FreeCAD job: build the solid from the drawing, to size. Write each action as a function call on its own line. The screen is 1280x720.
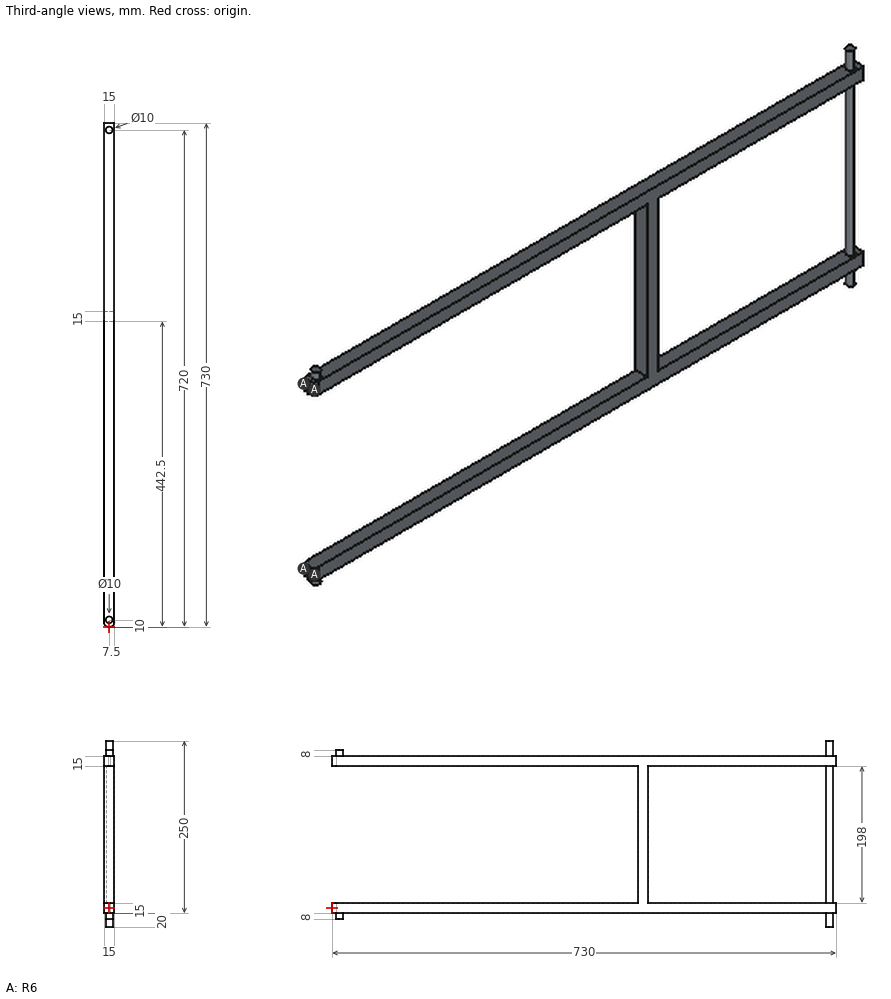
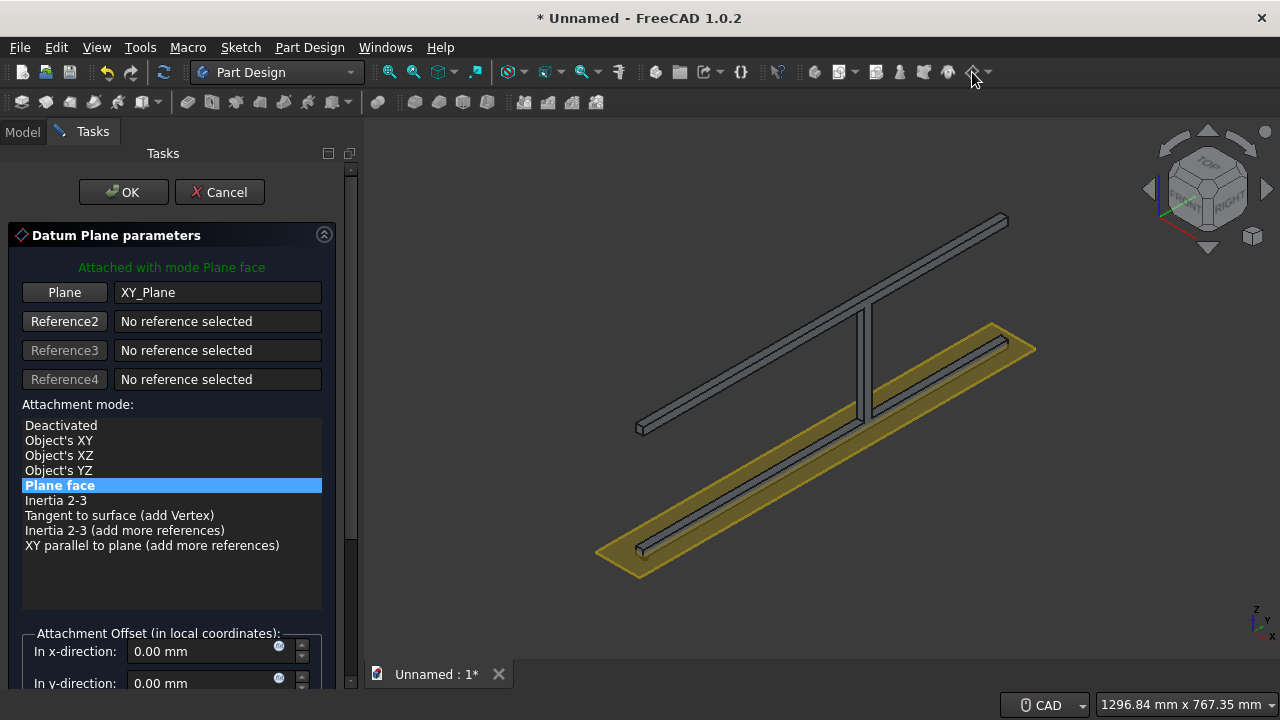
scroll(351, 426, down, 2)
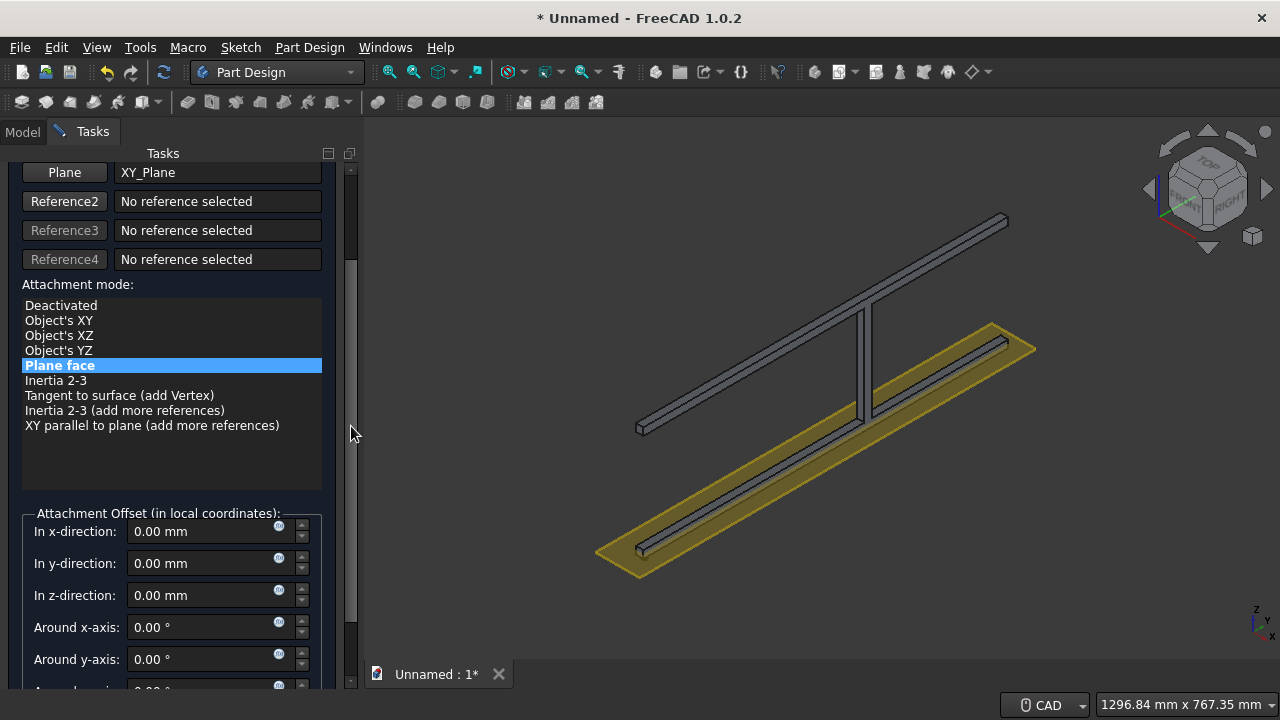
triple_click(210, 595)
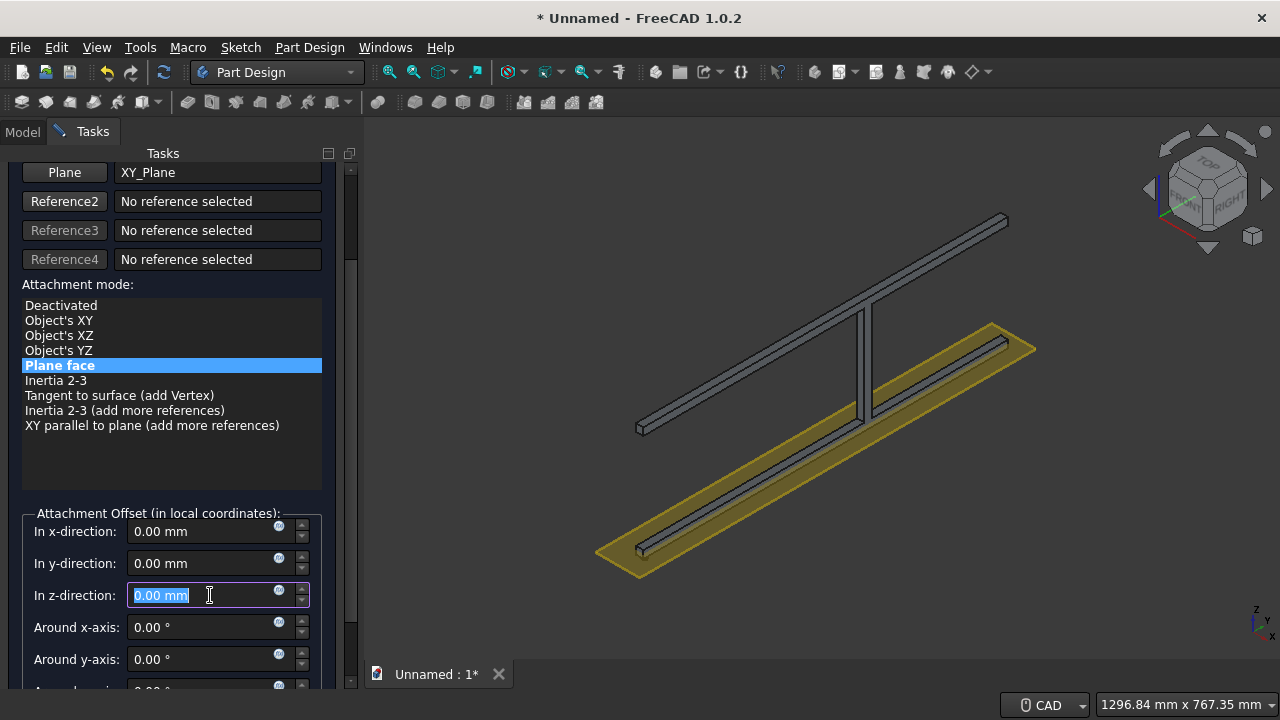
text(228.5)
key(Tab)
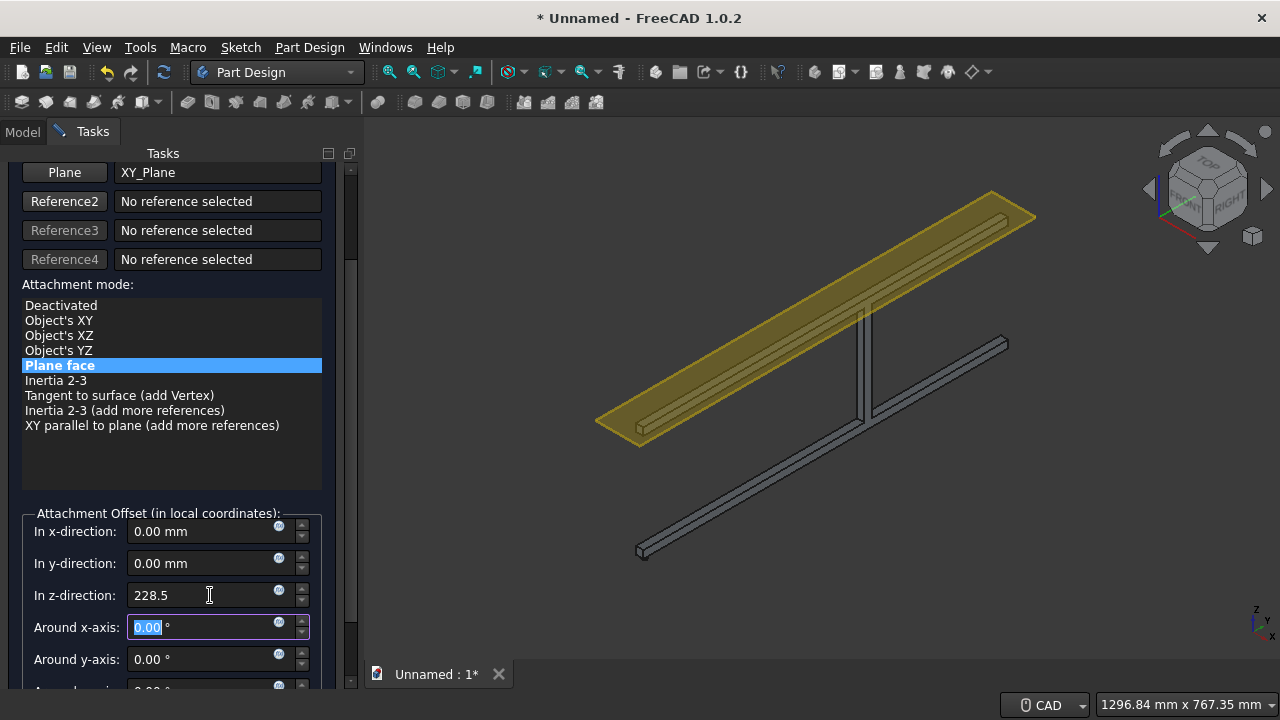
scroll(351, 426, up, 3)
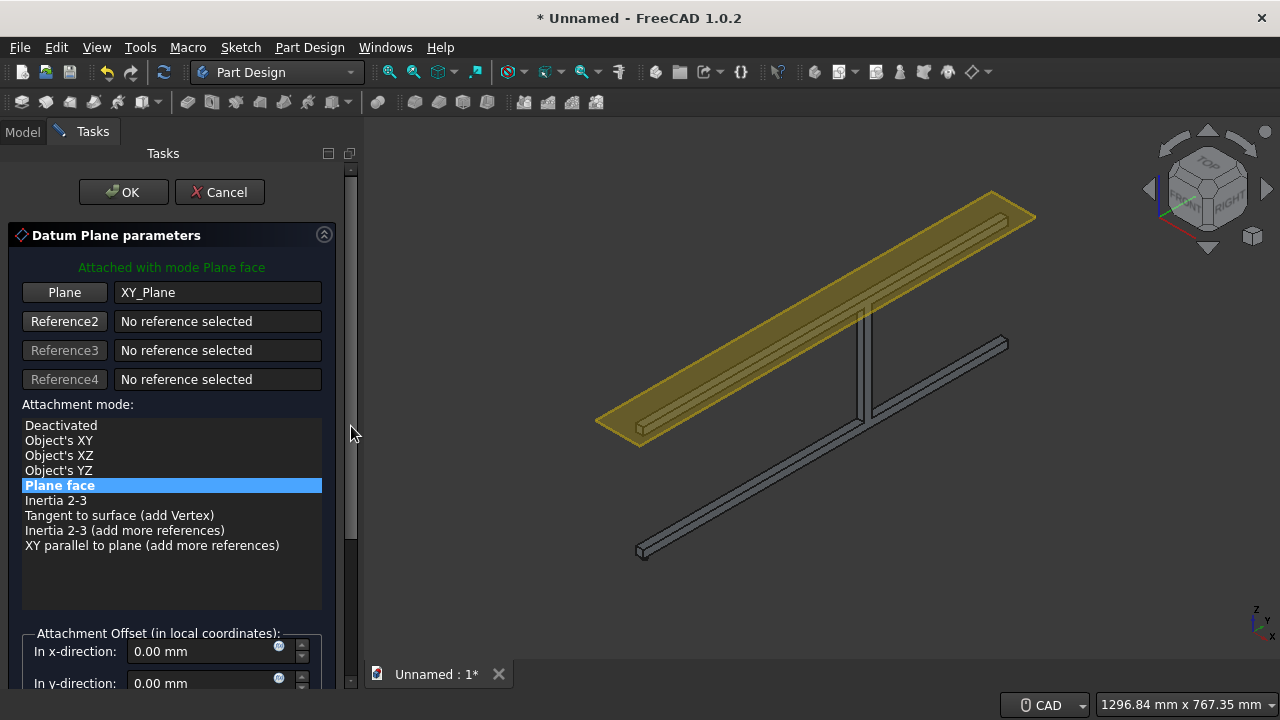
click(124, 192)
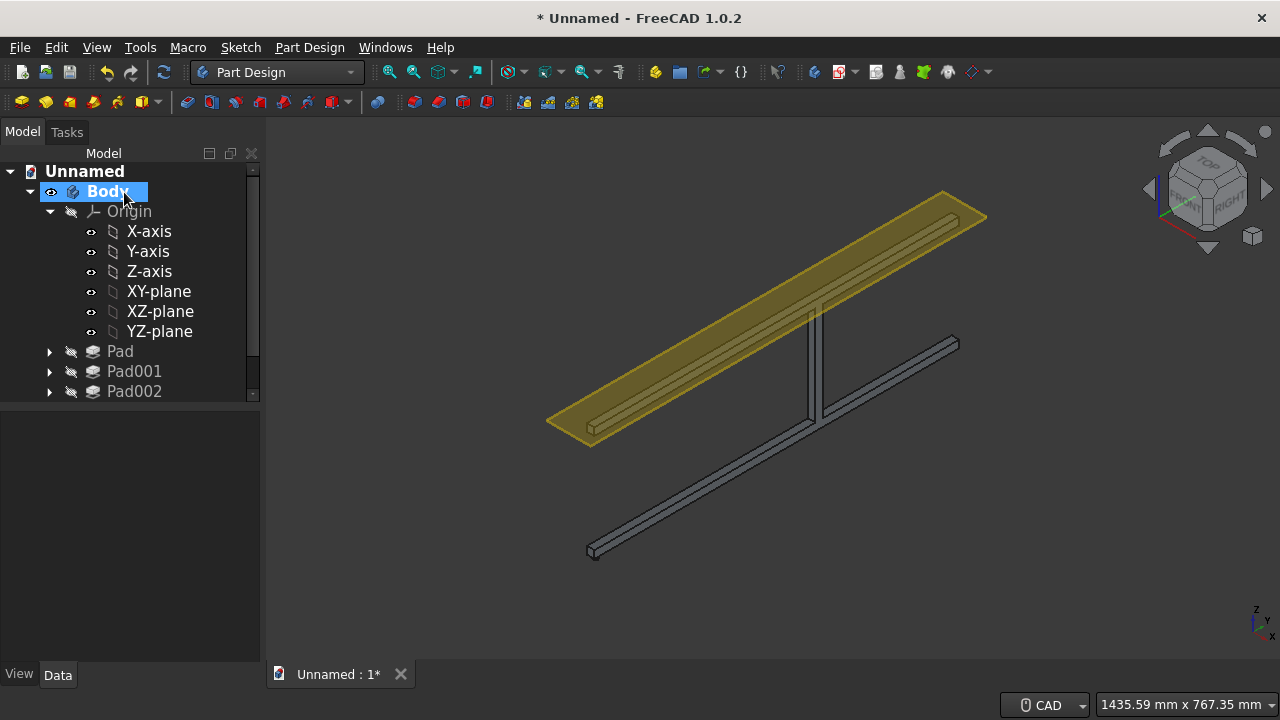
scroll(100, 287, down, 3)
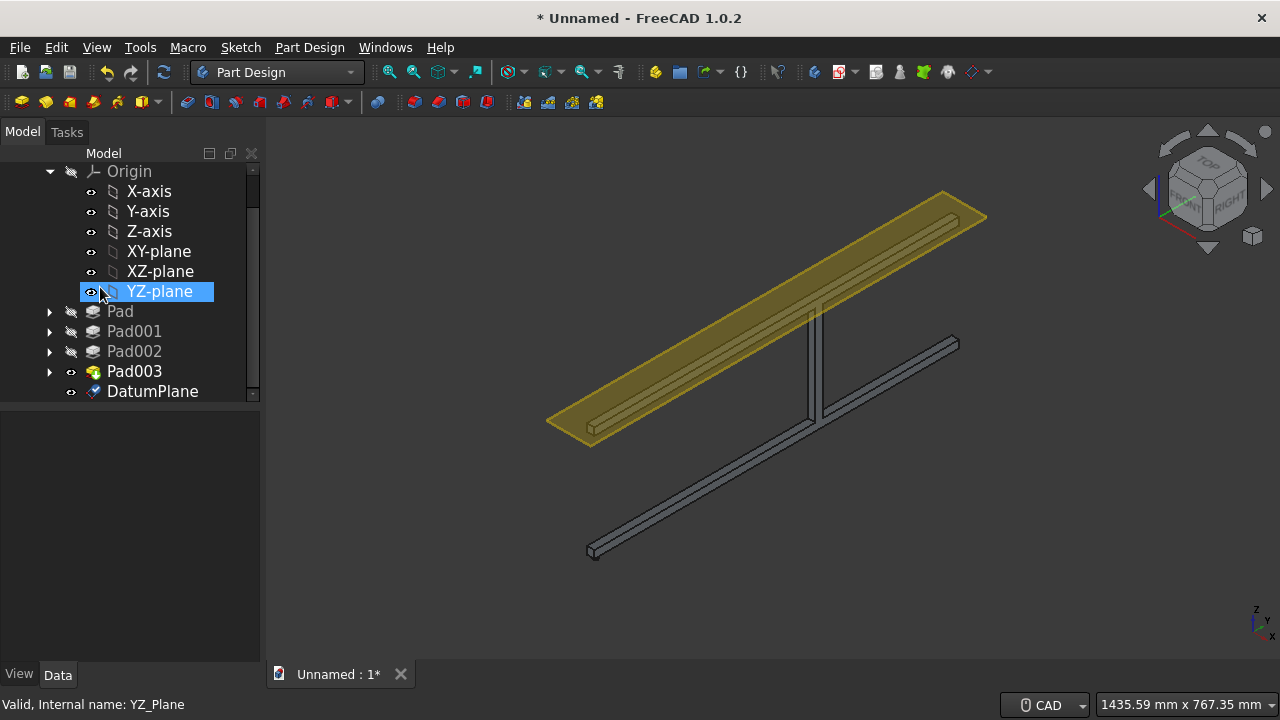
click(116, 392)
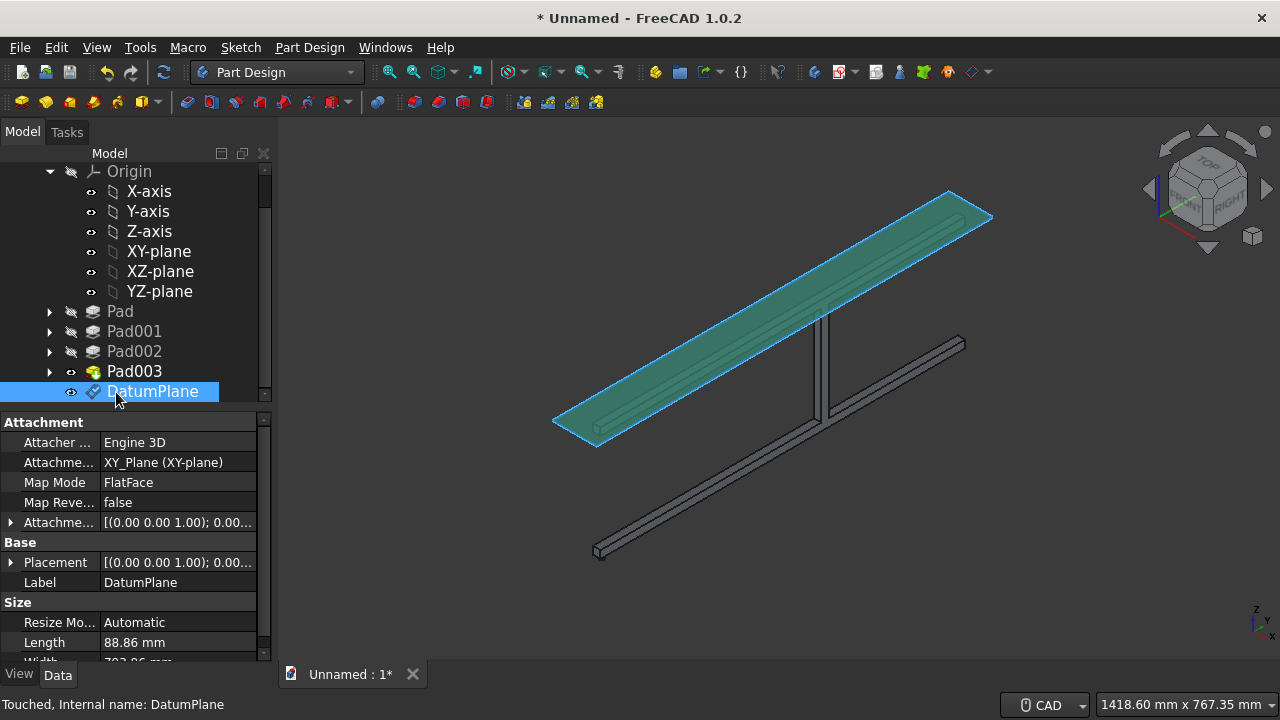
click(840, 72)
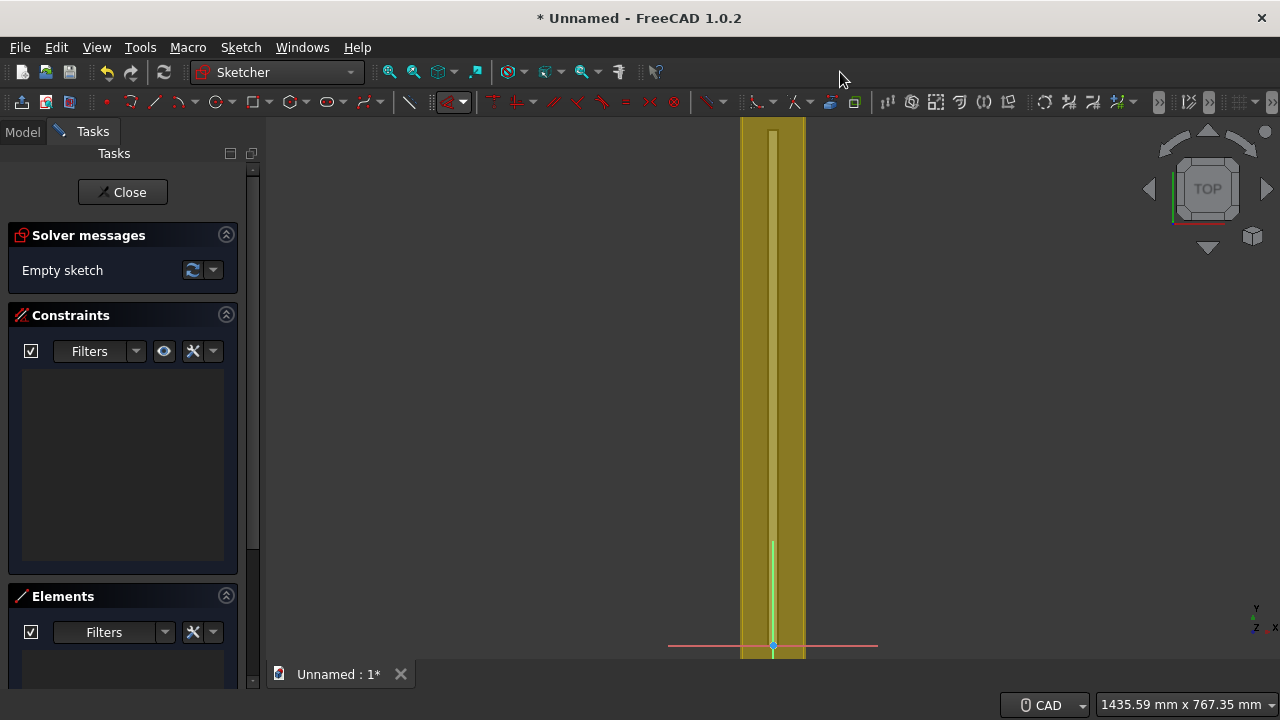
scroll(704, 388, down, 5)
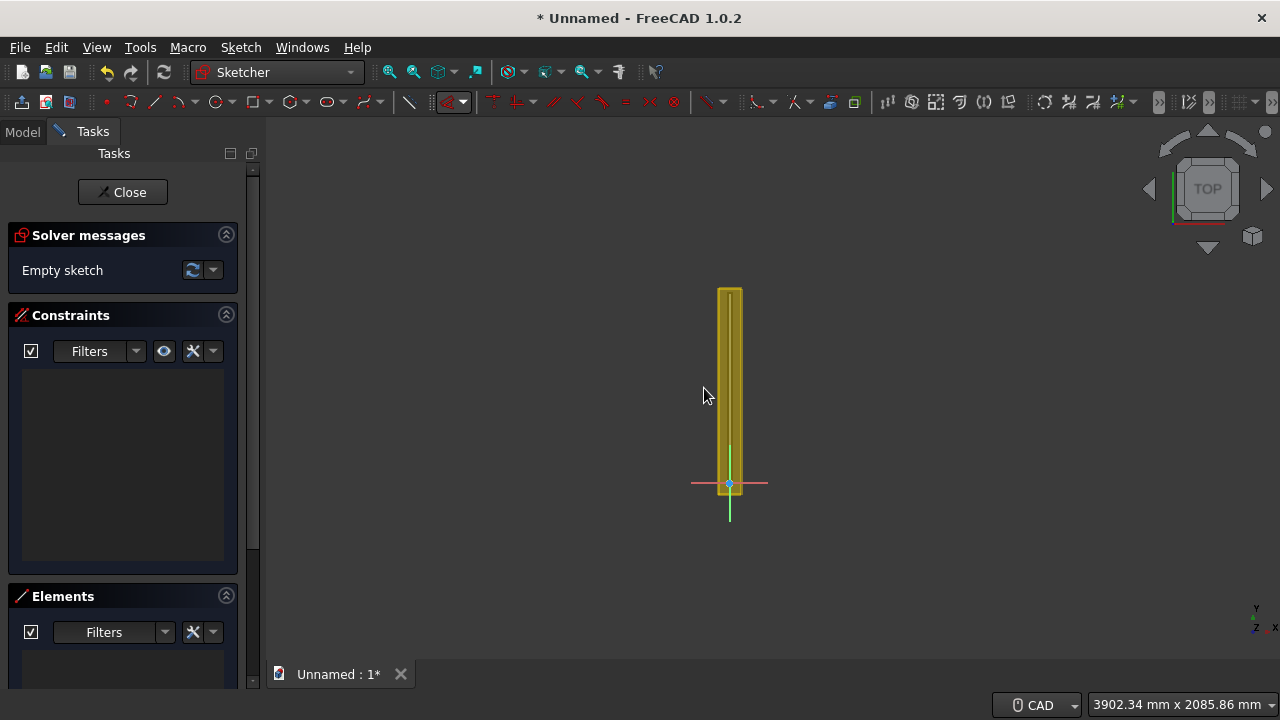
scroll(731, 486, up, 15)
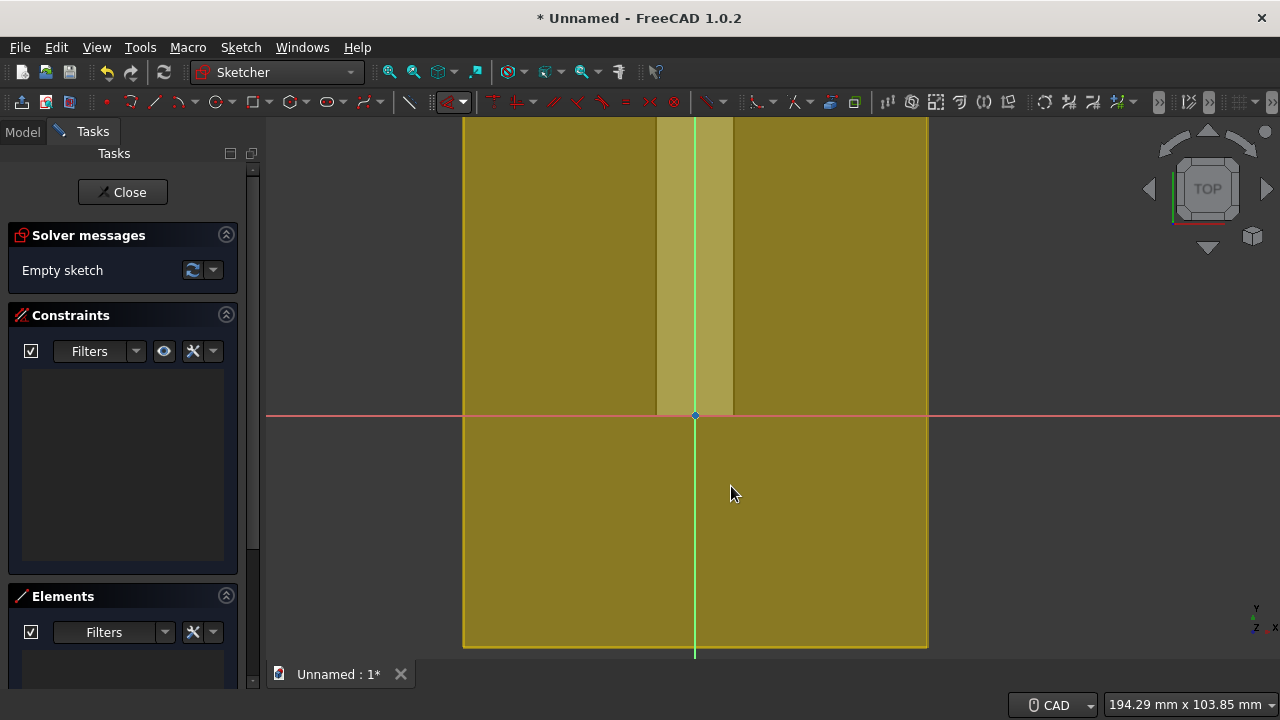
scroll(692, 373, up, 7)